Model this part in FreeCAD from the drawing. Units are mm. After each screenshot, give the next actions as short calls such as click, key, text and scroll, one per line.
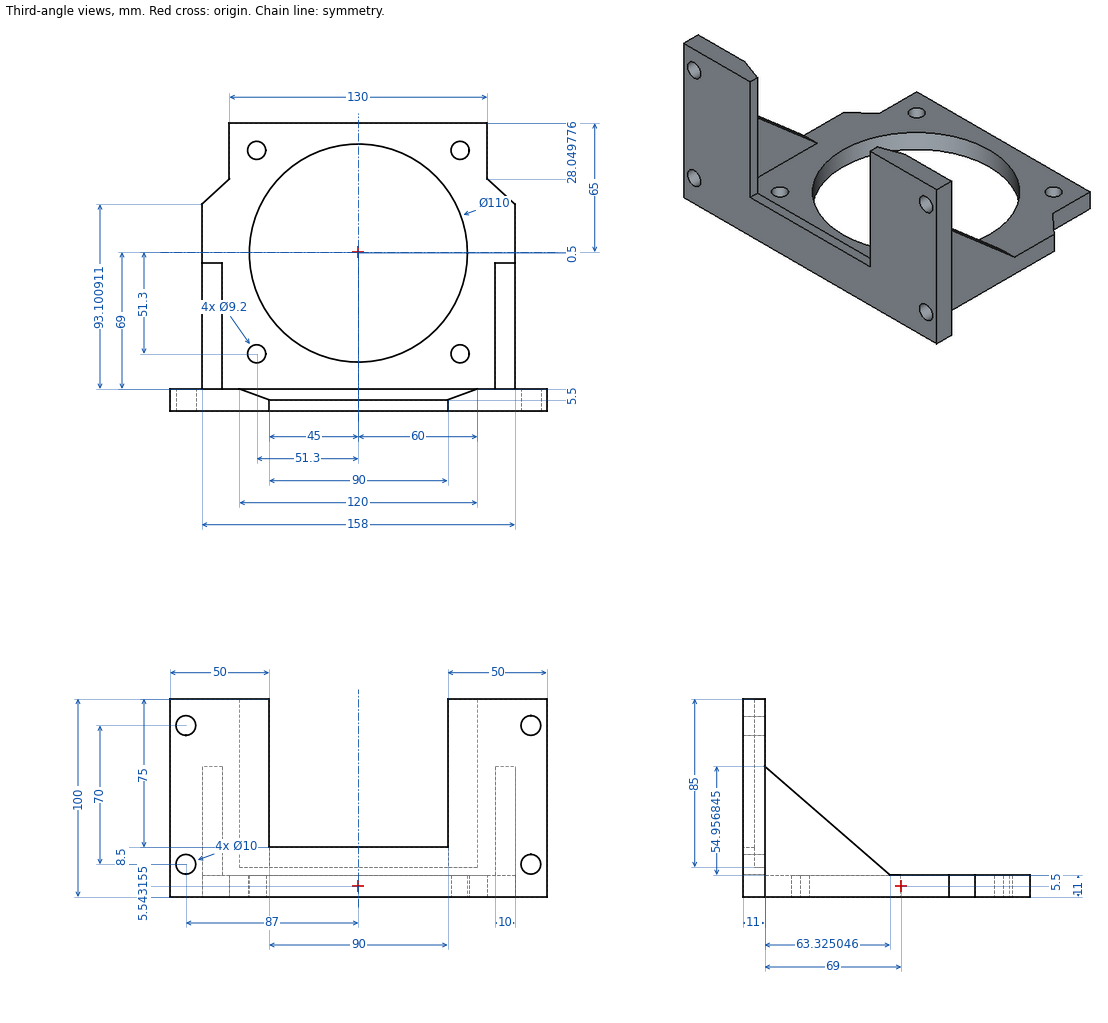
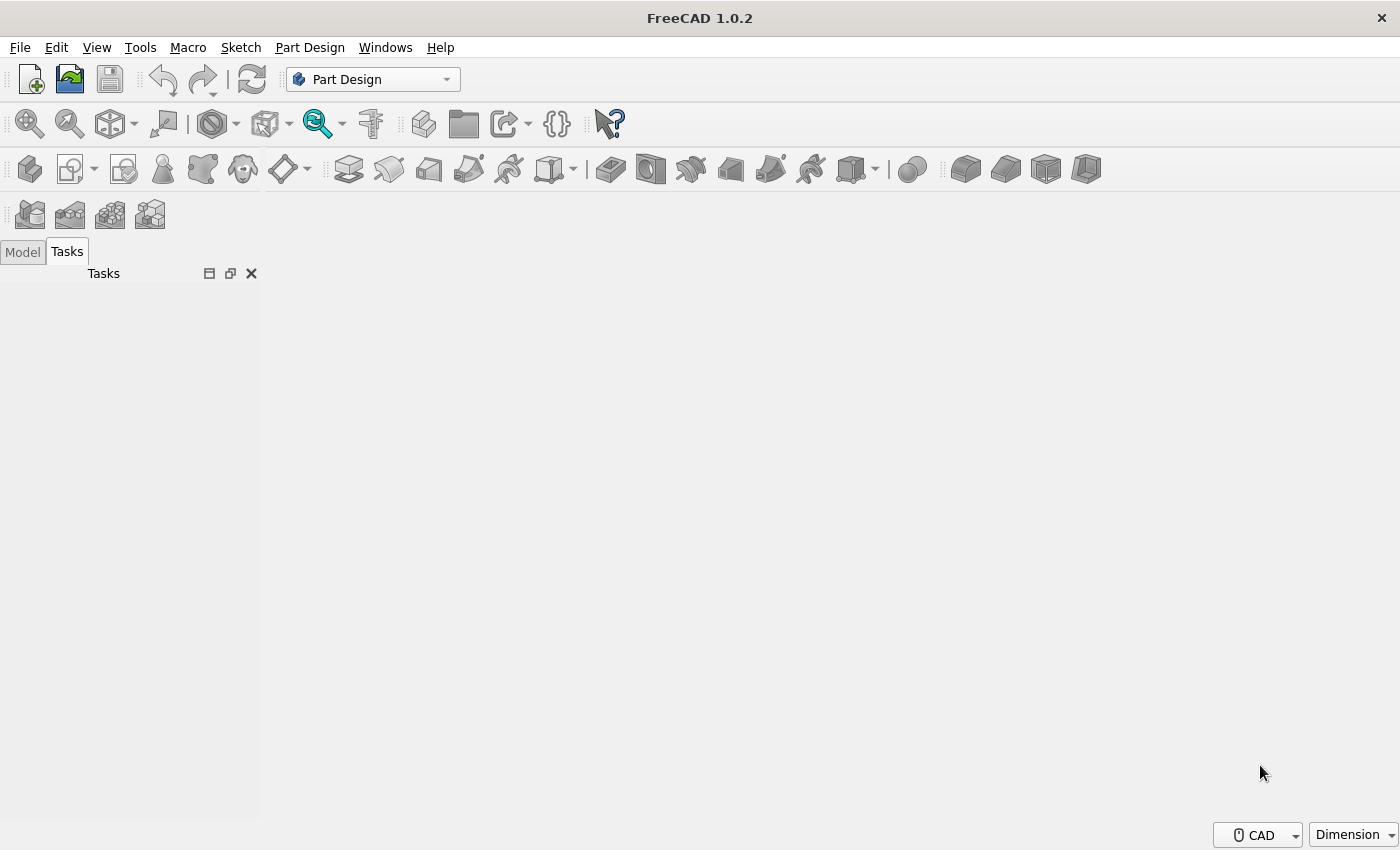
click(30, 80)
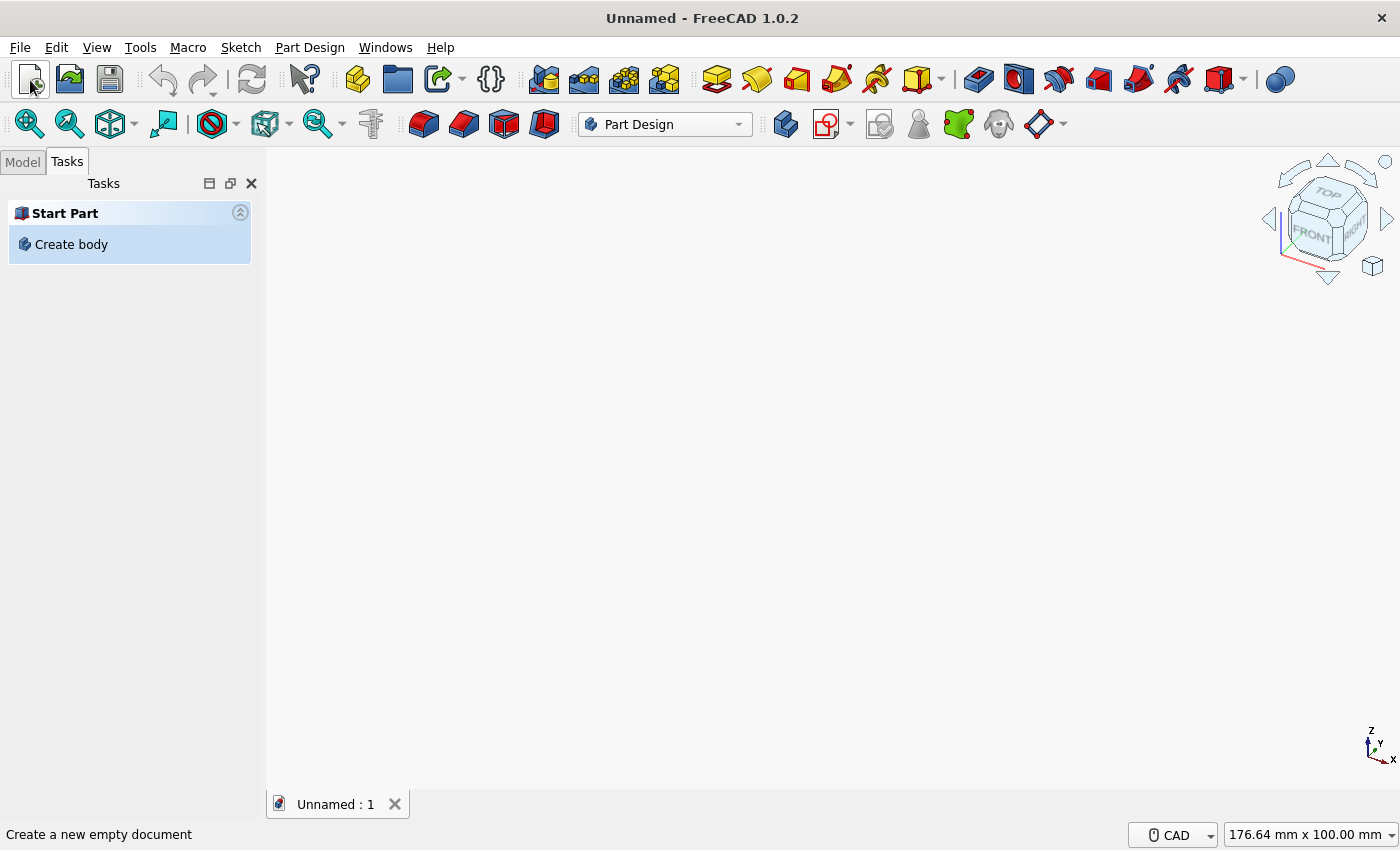
click(826, 124)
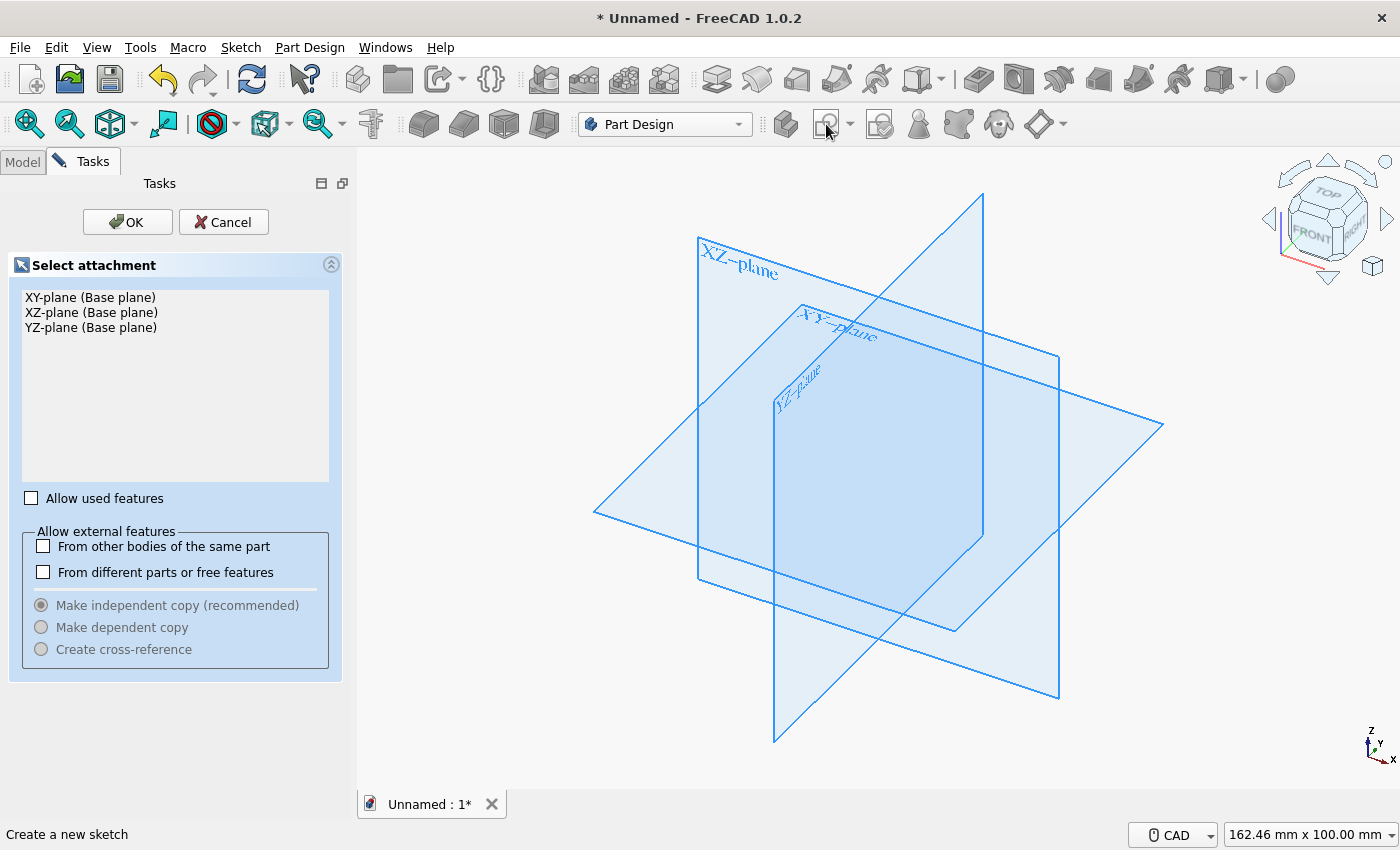
click(82, 298)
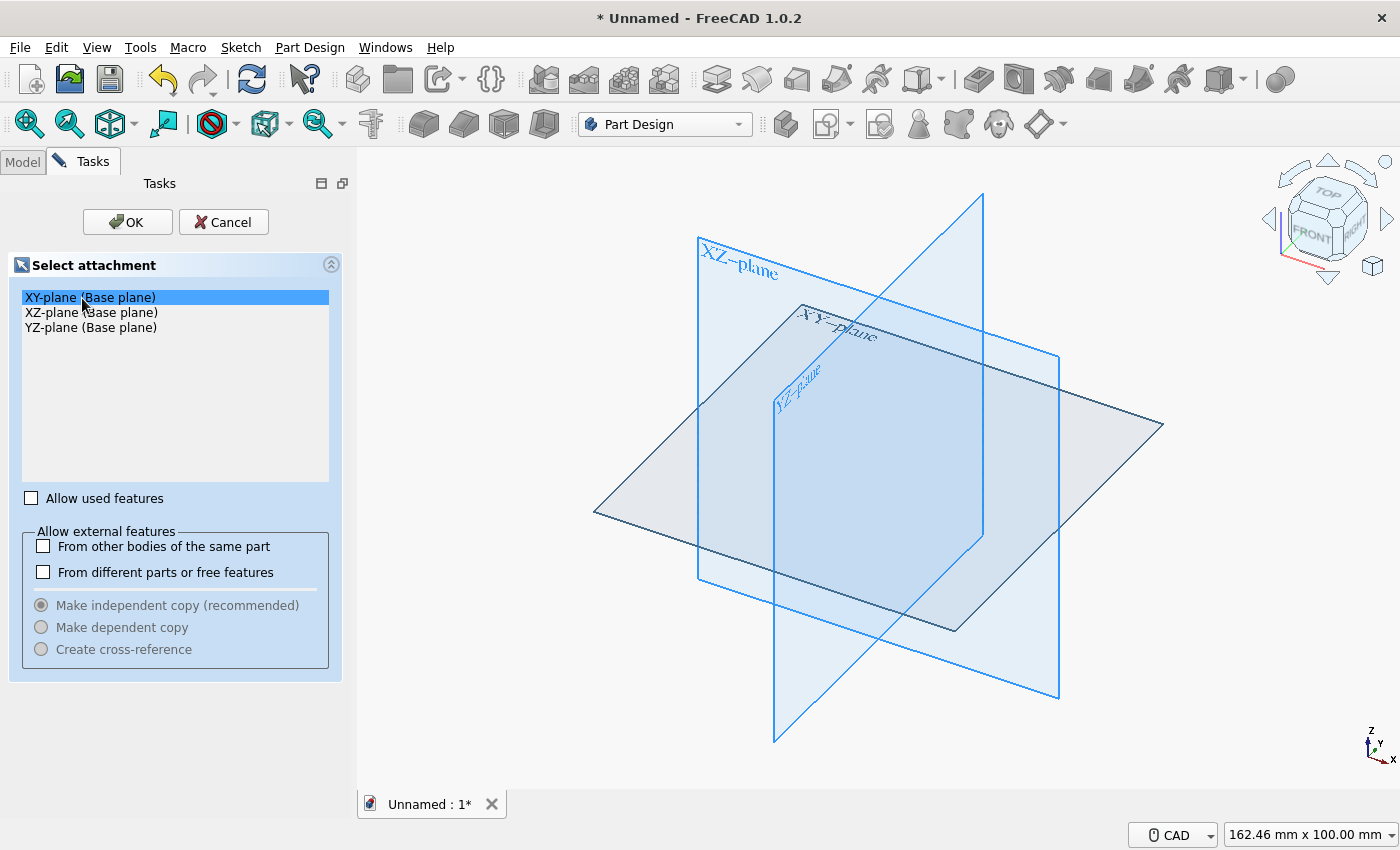
click(128, 222)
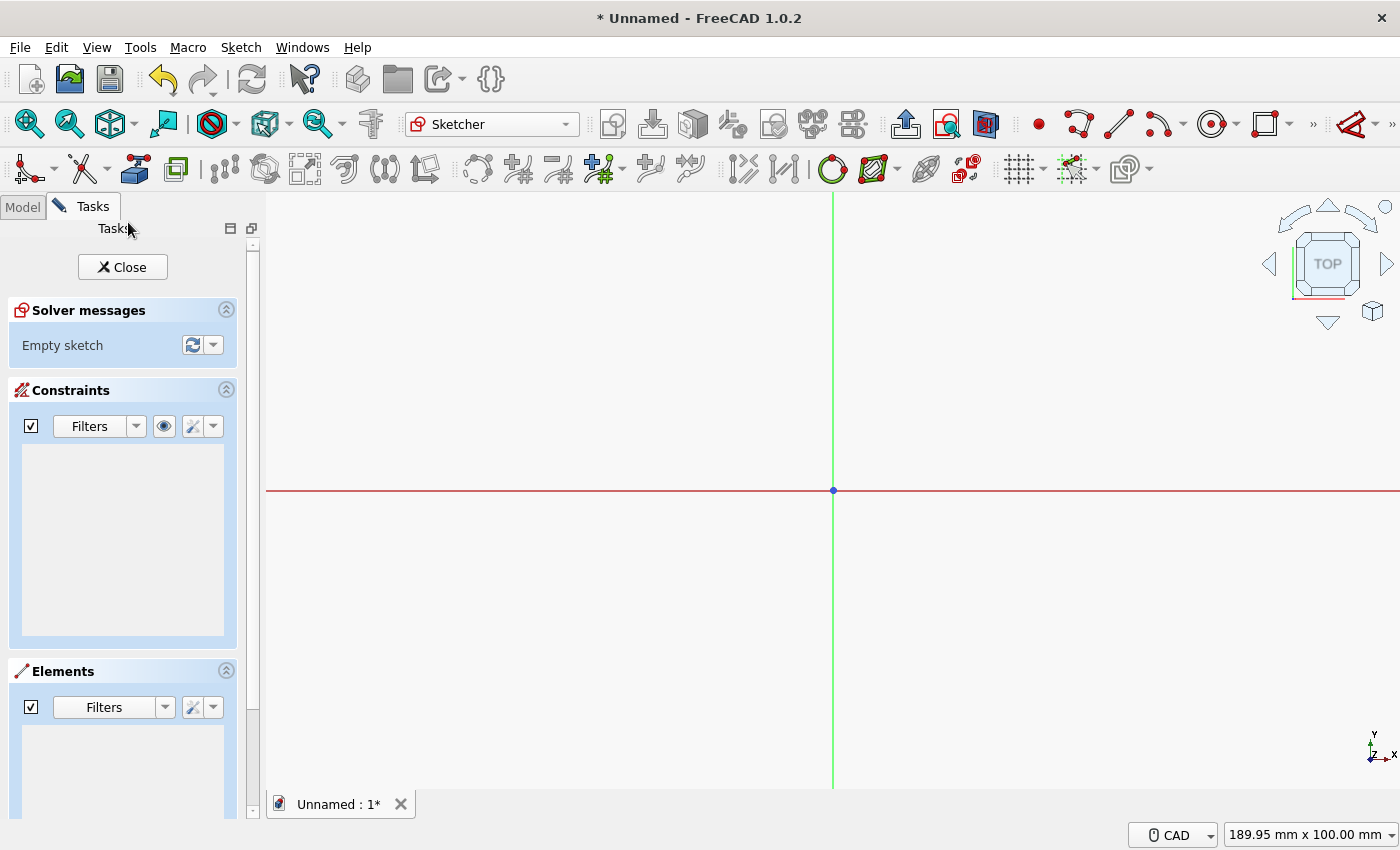
scroll(709, 481, down, 4)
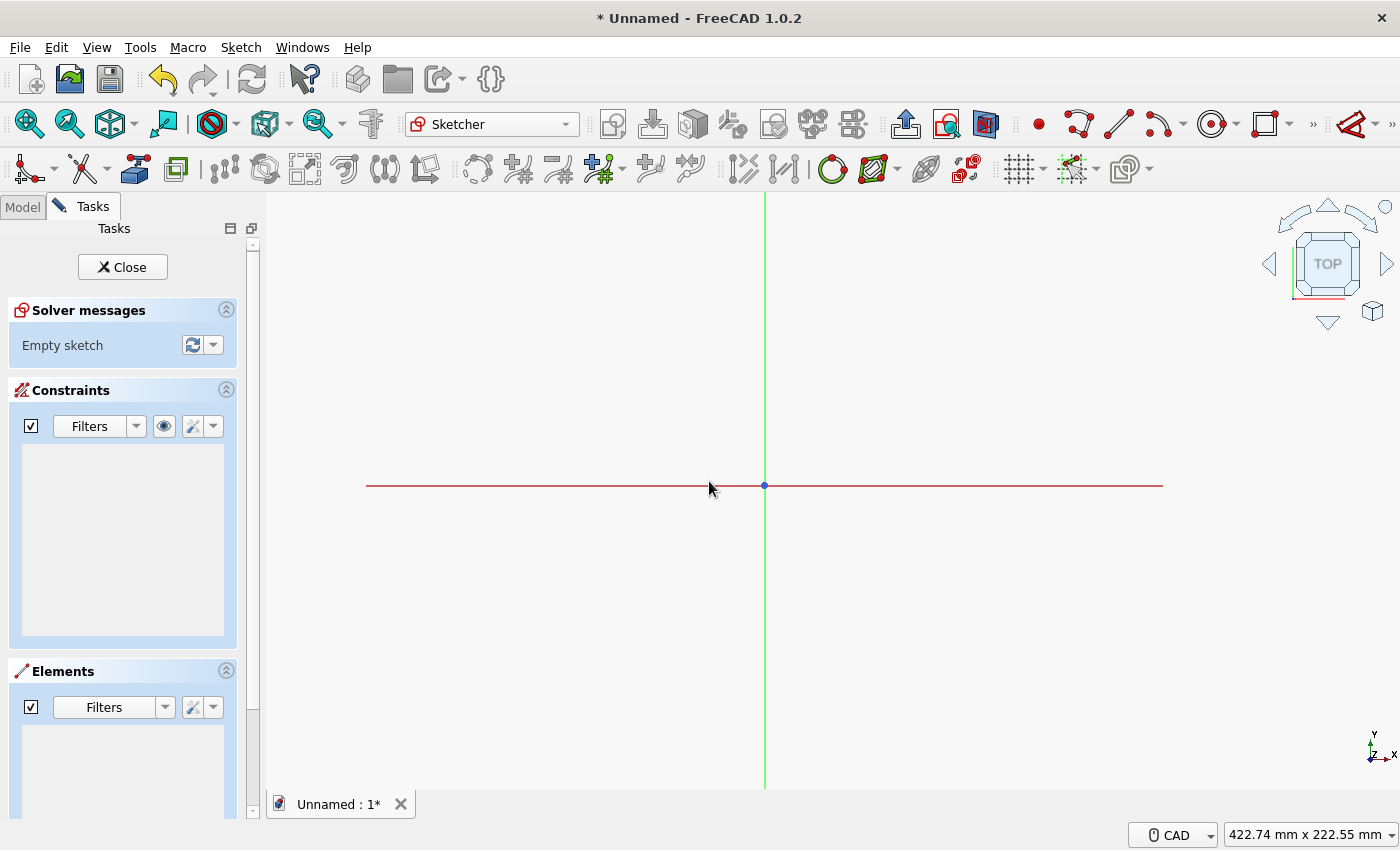
click(1080, 124)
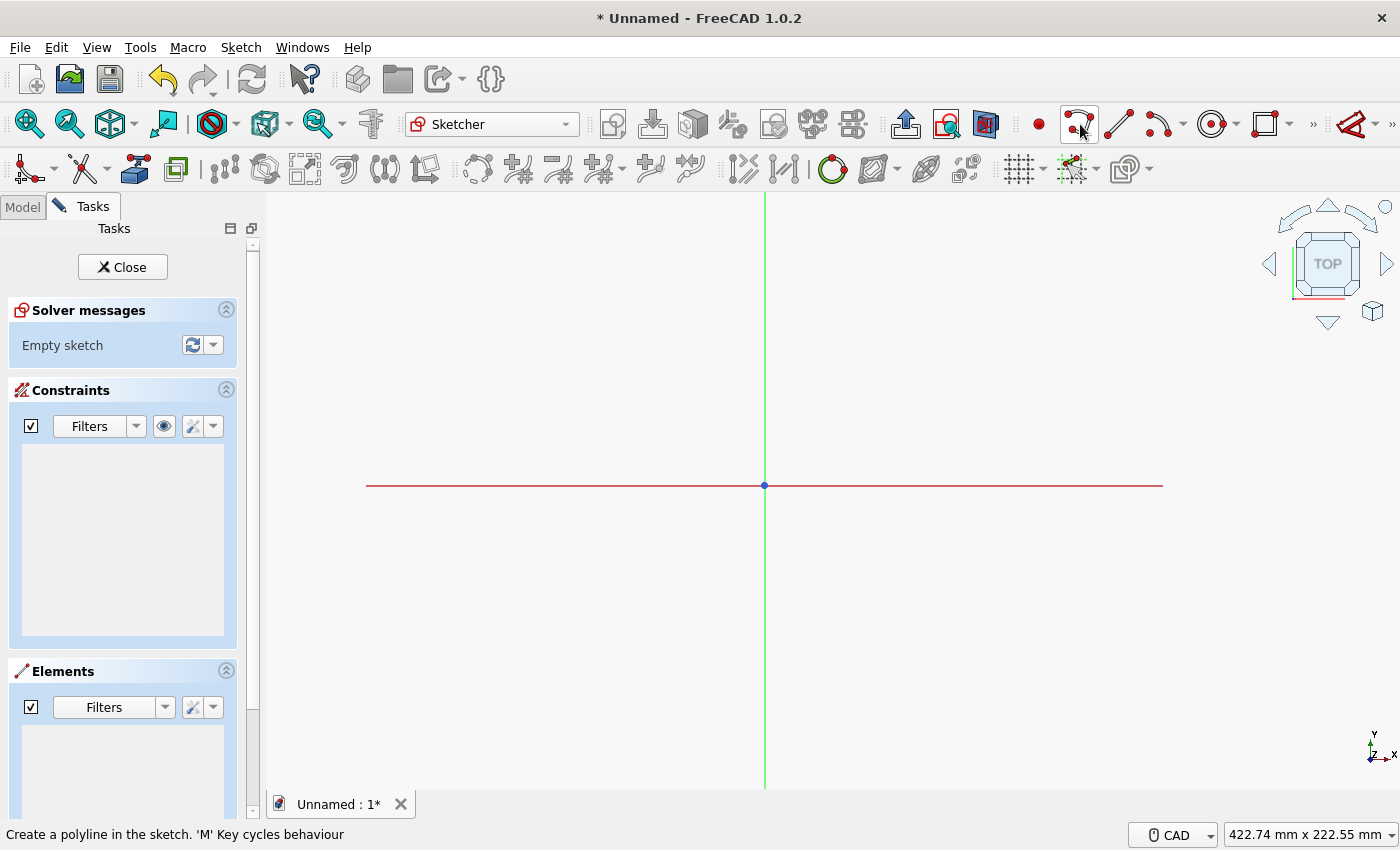
click(591, 386)
click(553, 421)
click(553, 671)
click(977, 671)
click(977, 421)
click(939, 386)
click(939, 311)
click(591, 311)
click(591, 387)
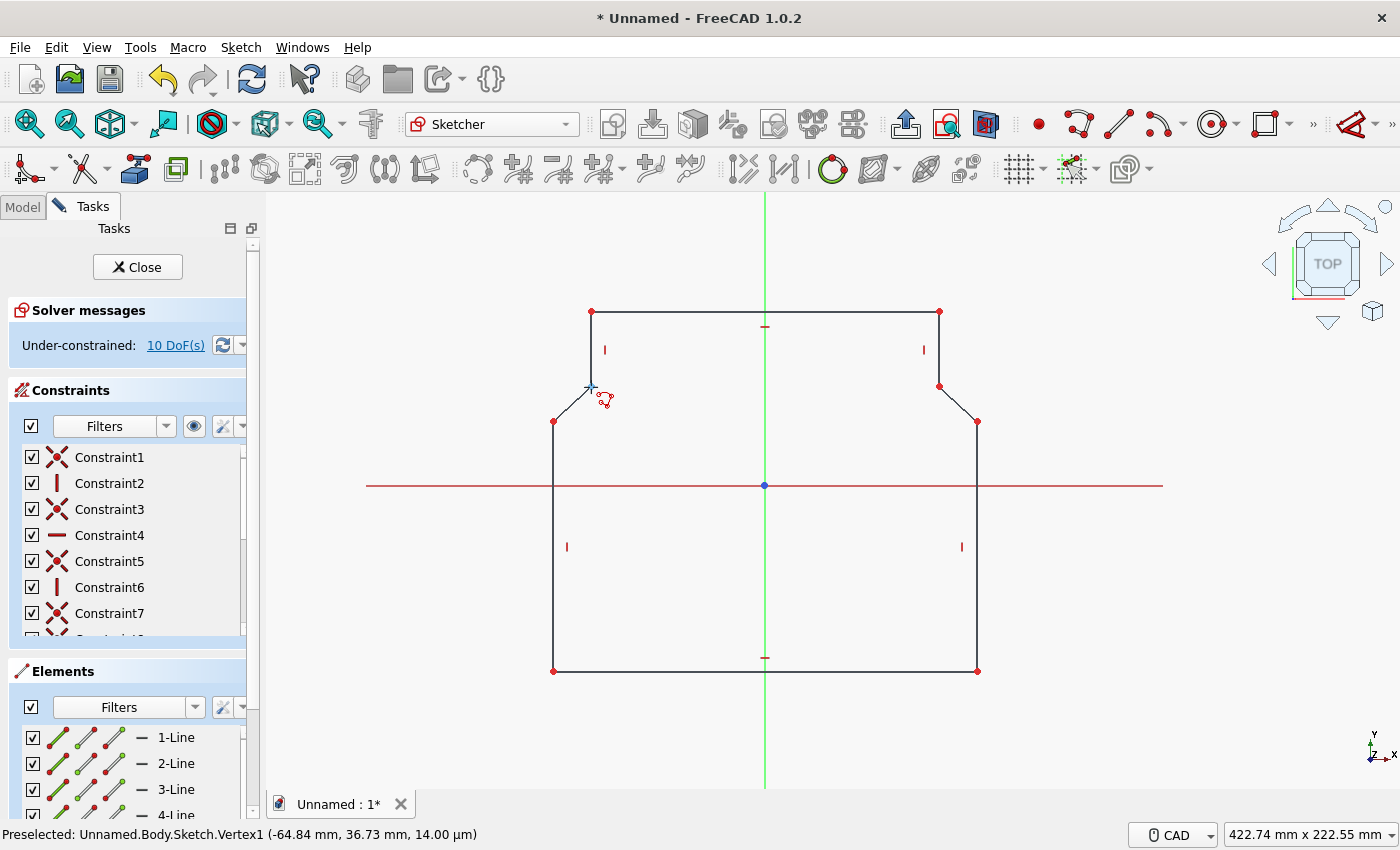
click(1212, 124)